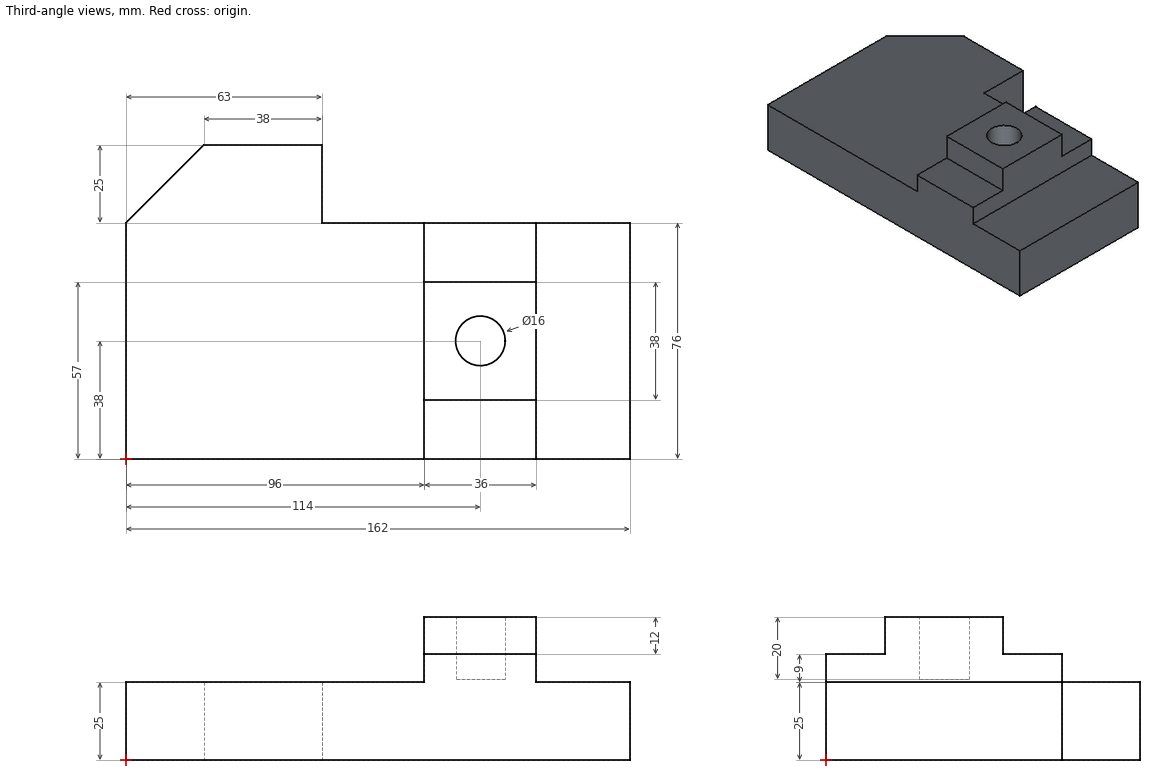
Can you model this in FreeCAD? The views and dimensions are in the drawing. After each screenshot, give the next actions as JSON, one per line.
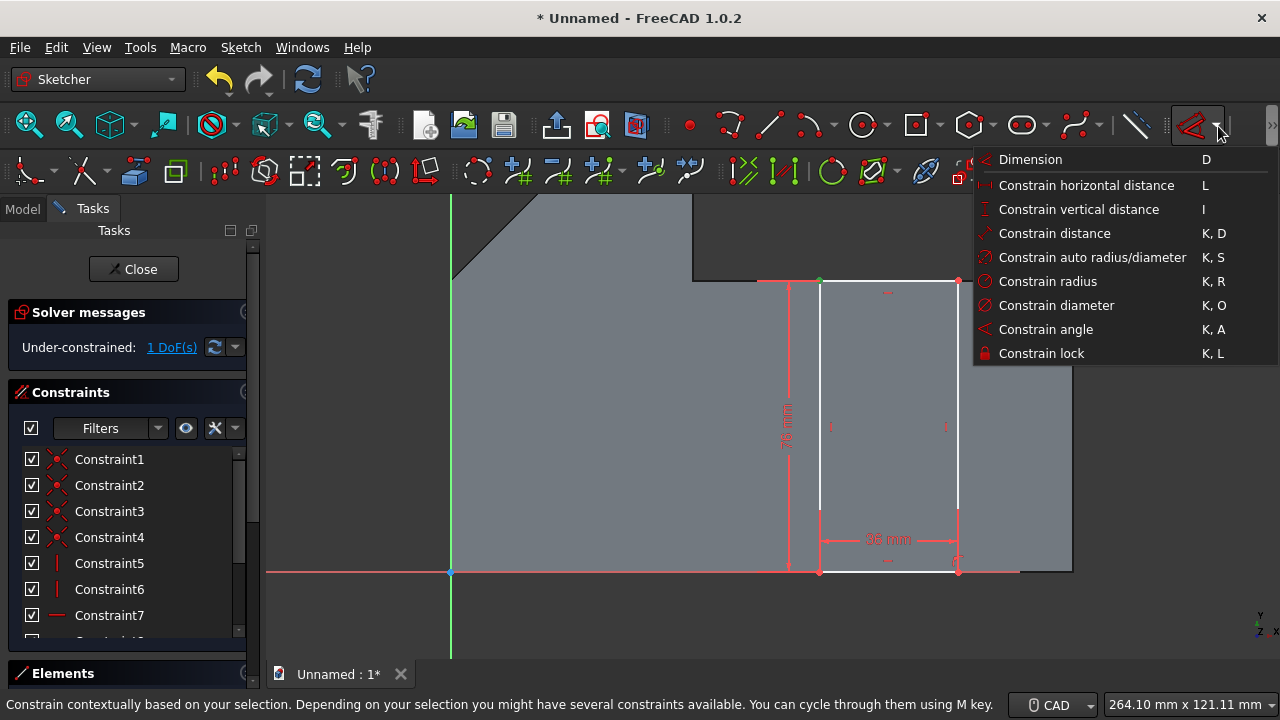
{"action": "left_click", "coordinate": [1126, 185]}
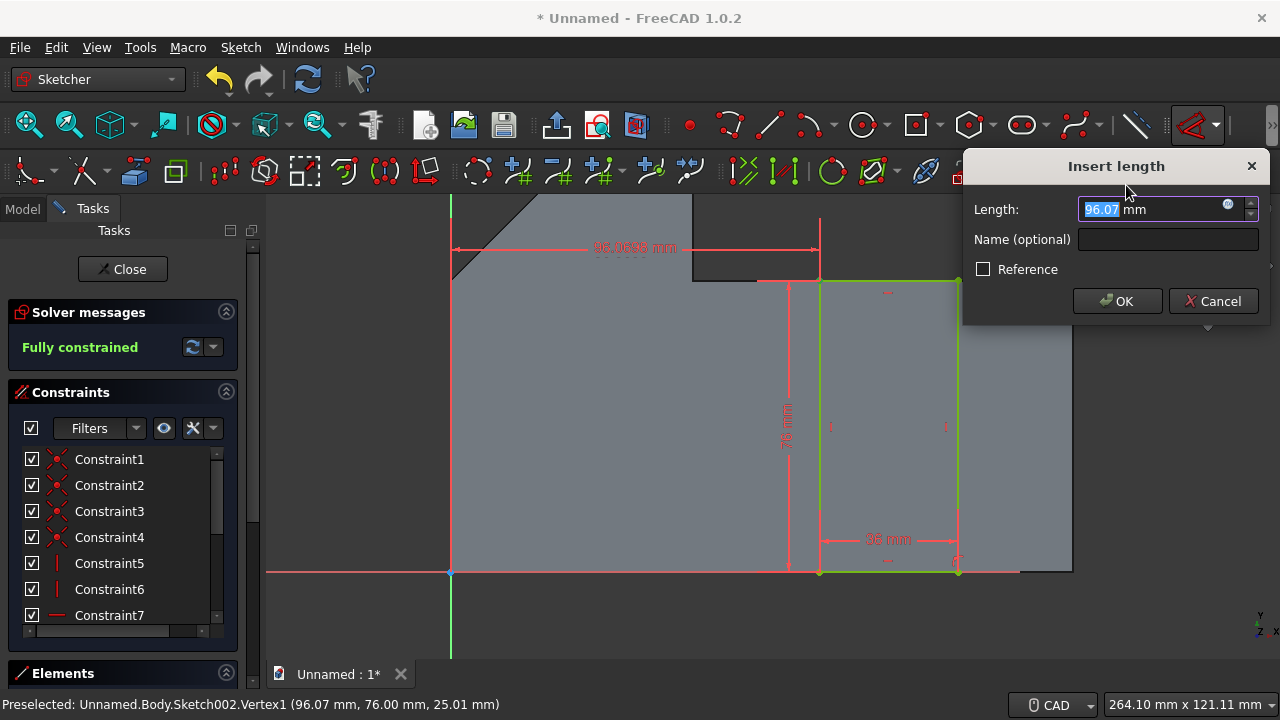
{"action": "type", "text": "96"}
{"action": "key", "text": "Return"}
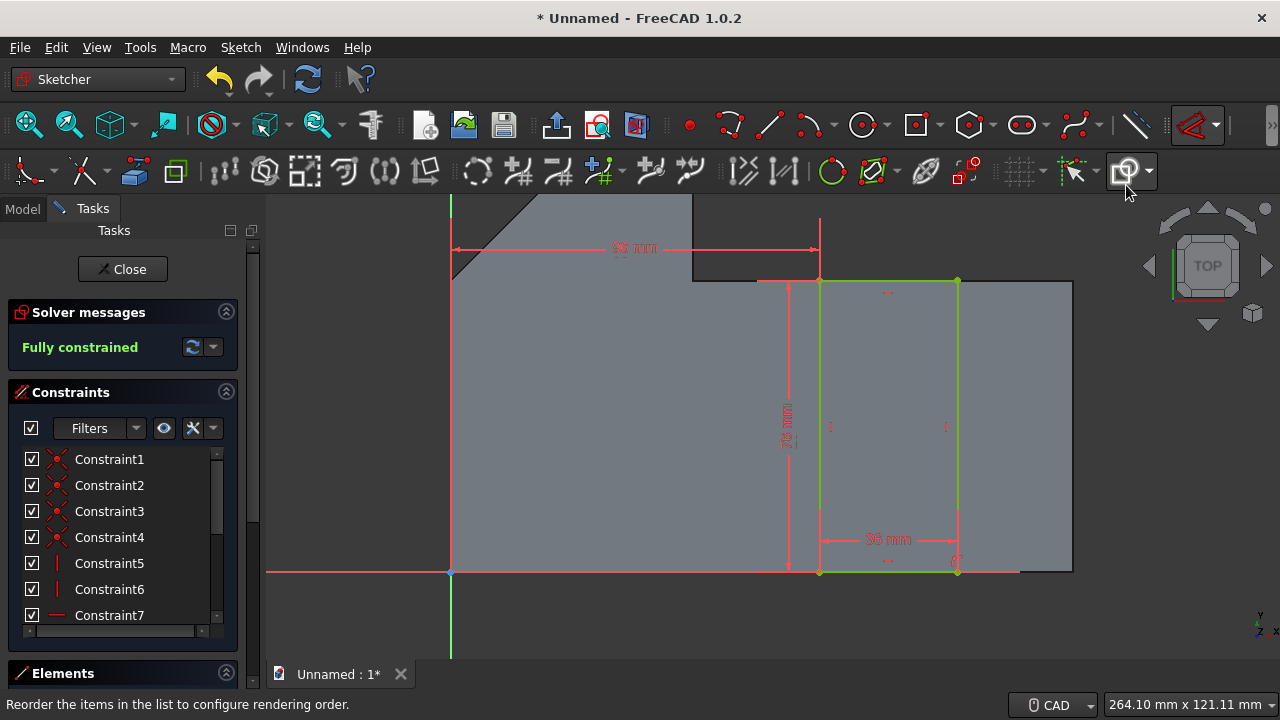
{"action": "left_click", "coordinate": [123, 269]}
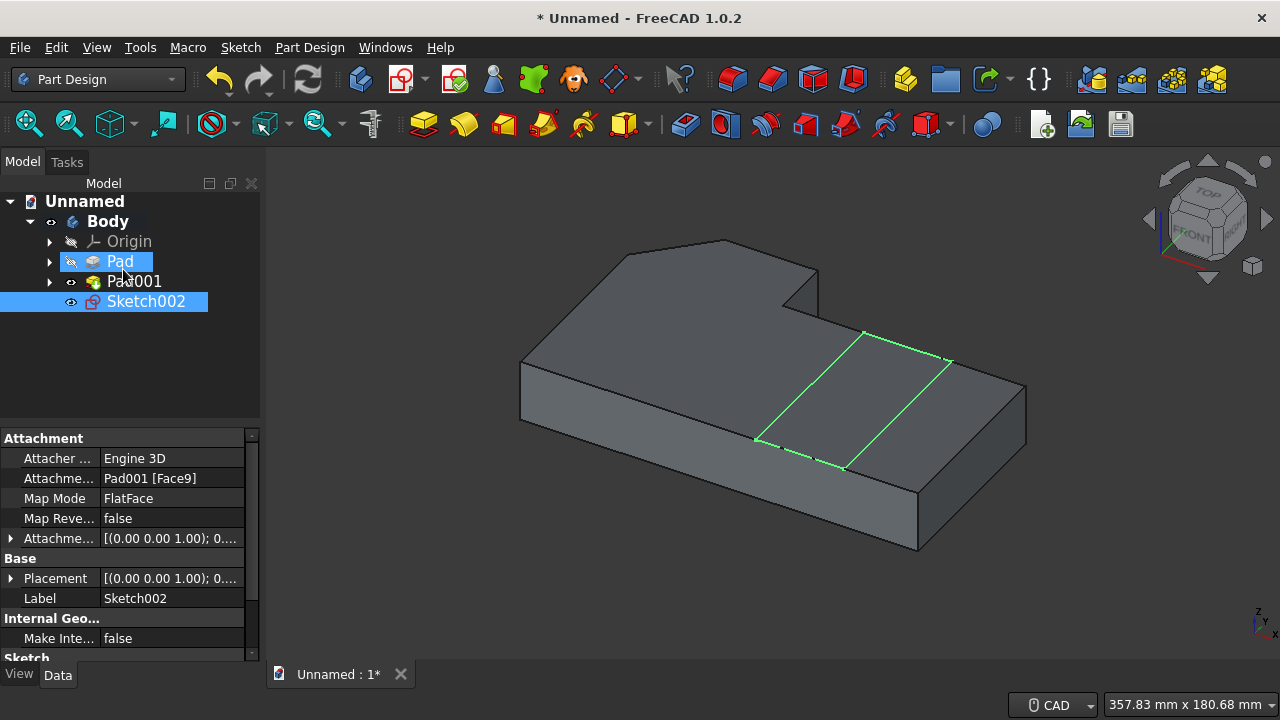
{"action": "left_click", "coordinate": [424, 124]}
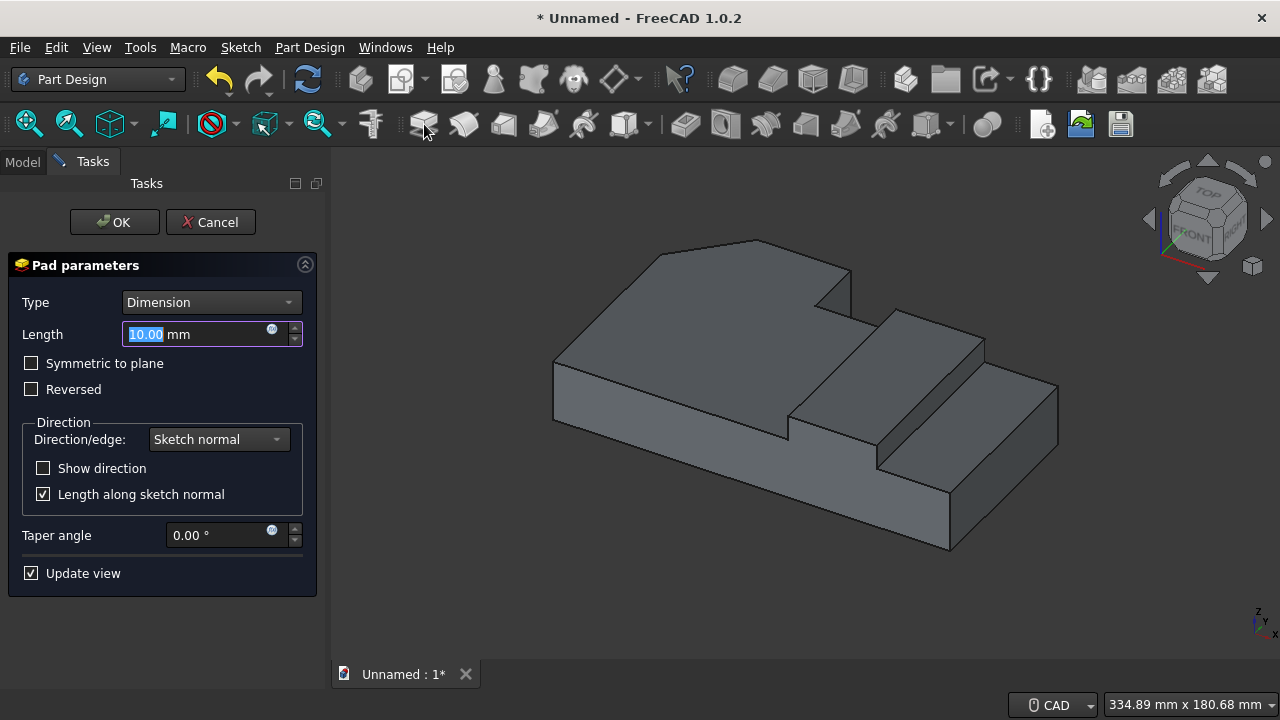
{"action": "type", "text": "9"}
{"action": "key", "text": "Tab"}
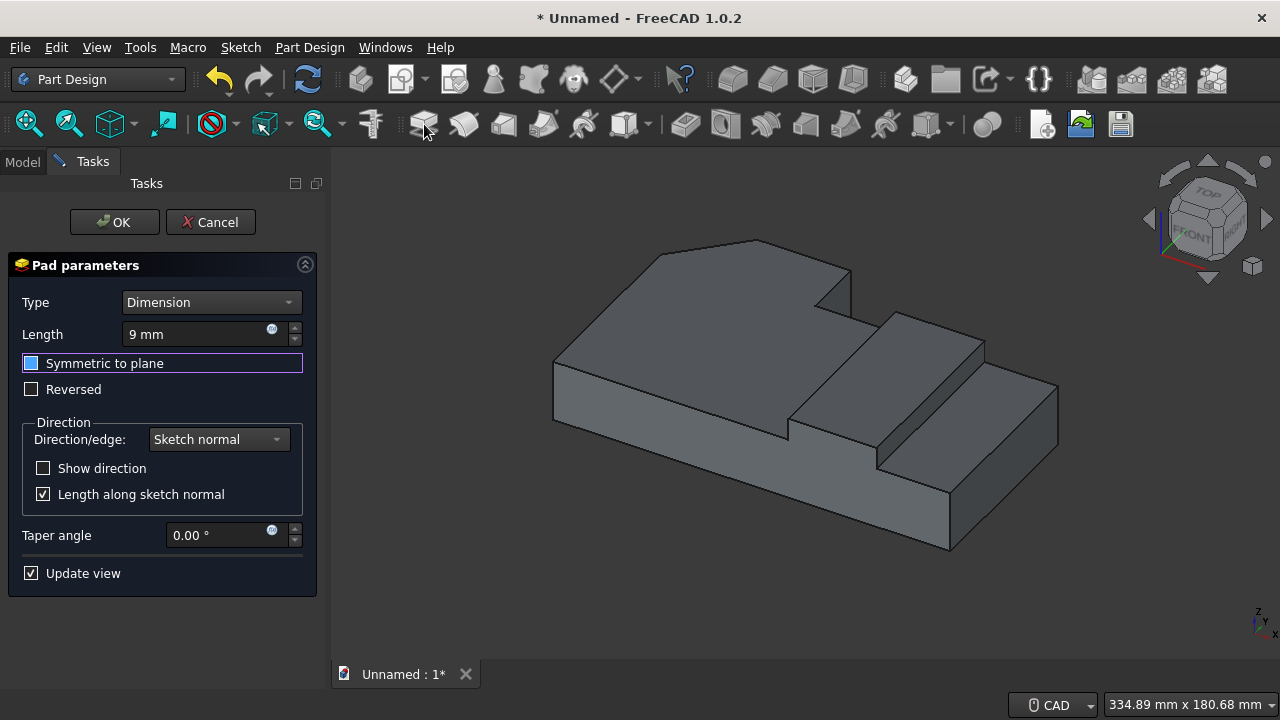
{"action": "left_click", "coordinate": [115, 222]}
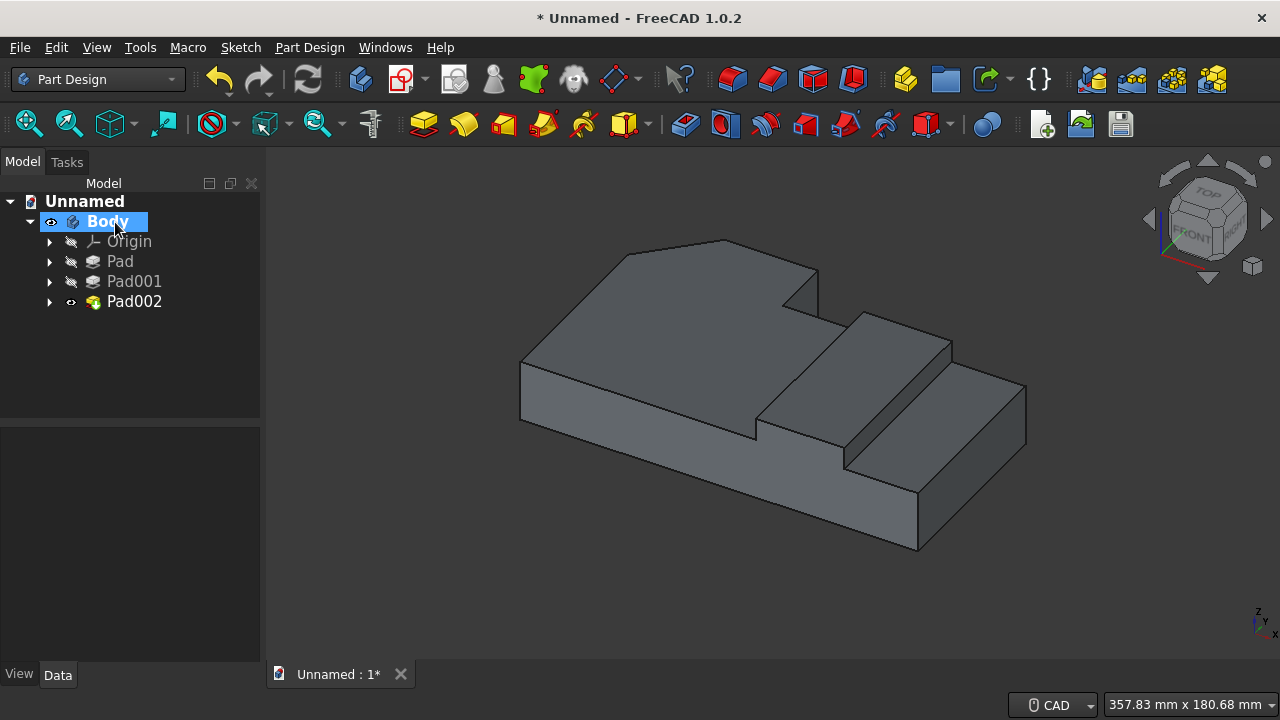
{"action": "left_click", "coordinate": [869, 364]}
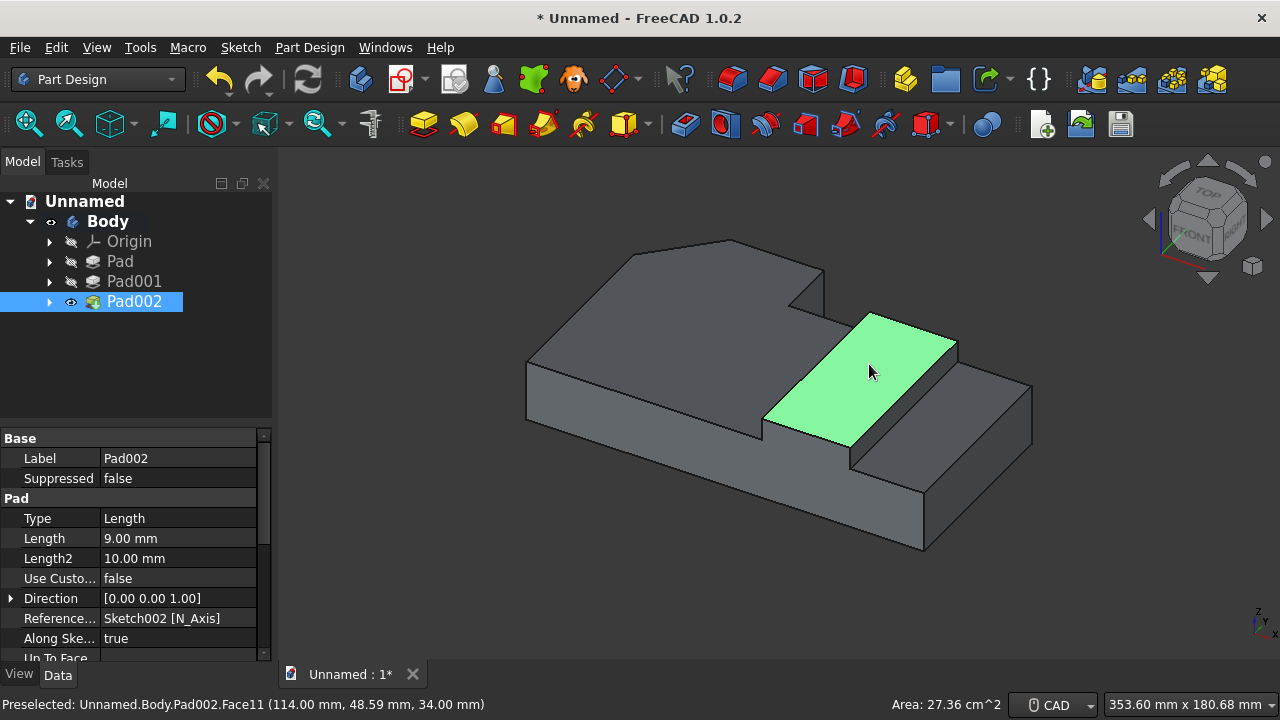
{"action": "left_click", "coordinate": [402, 80]}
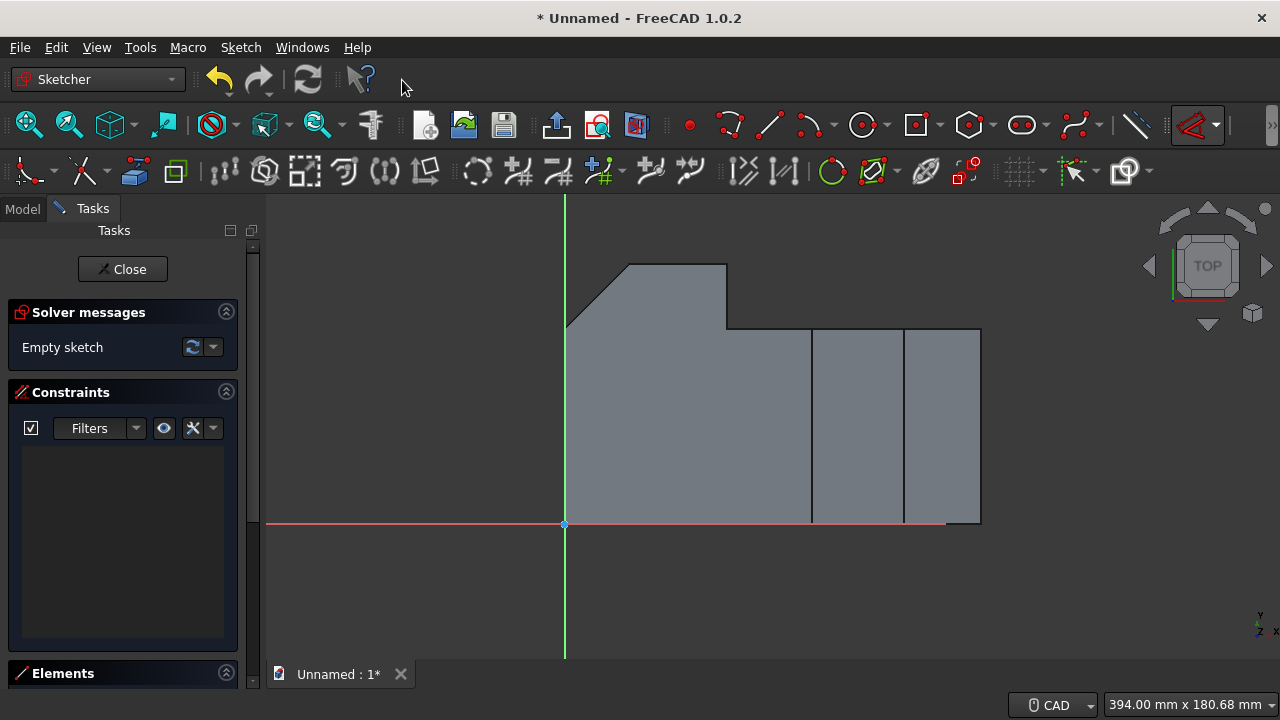
{"action": "scroll", "coordinate": [947, 426], "scroll_direction": "up", "scroll_amount": 5}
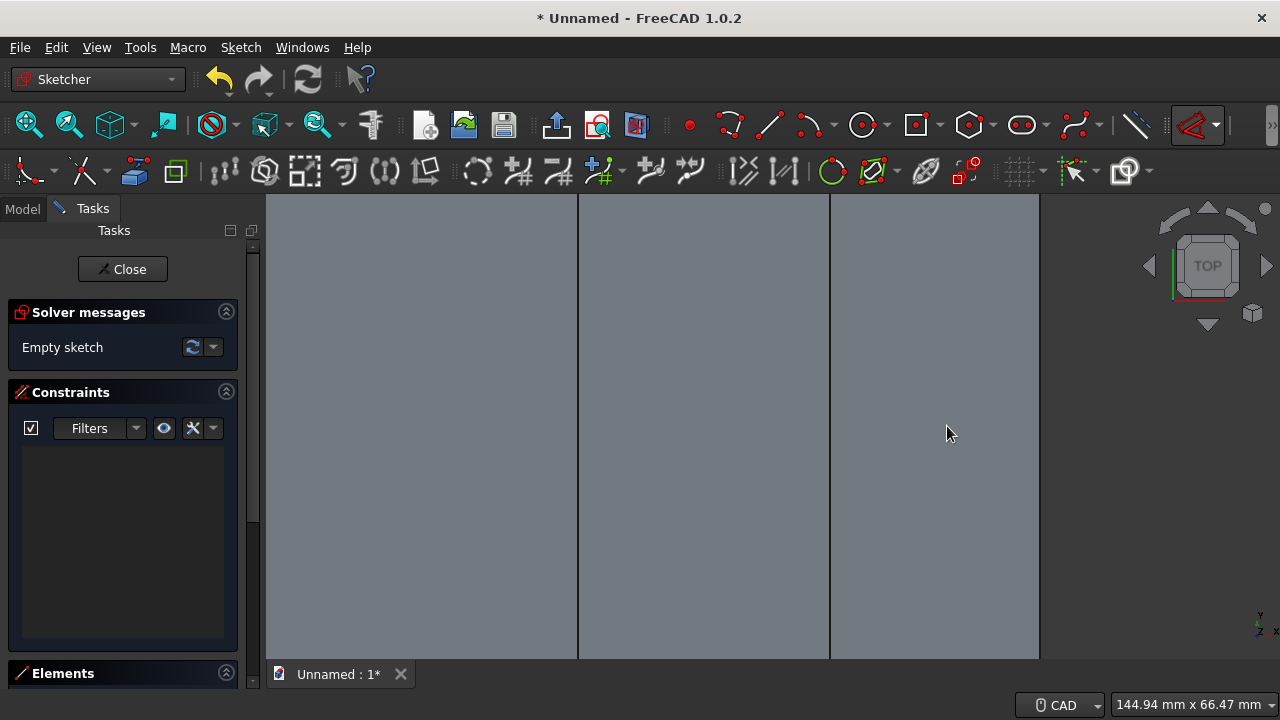
{"action": "key", "text": "g r"}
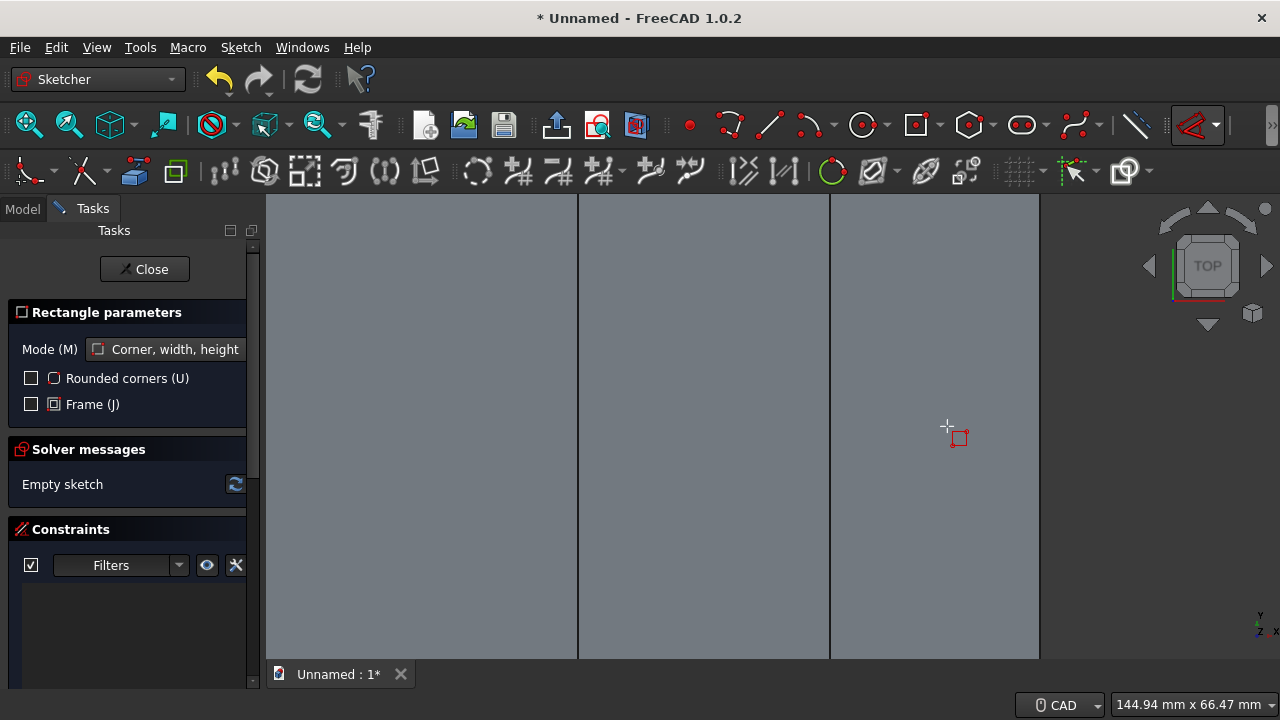
{"action": "left_click", "coordinate": [578, 294]}
{"action": "left_click", "coordinate": [830, 559]}
{"action": "key", "text": "Escape"}